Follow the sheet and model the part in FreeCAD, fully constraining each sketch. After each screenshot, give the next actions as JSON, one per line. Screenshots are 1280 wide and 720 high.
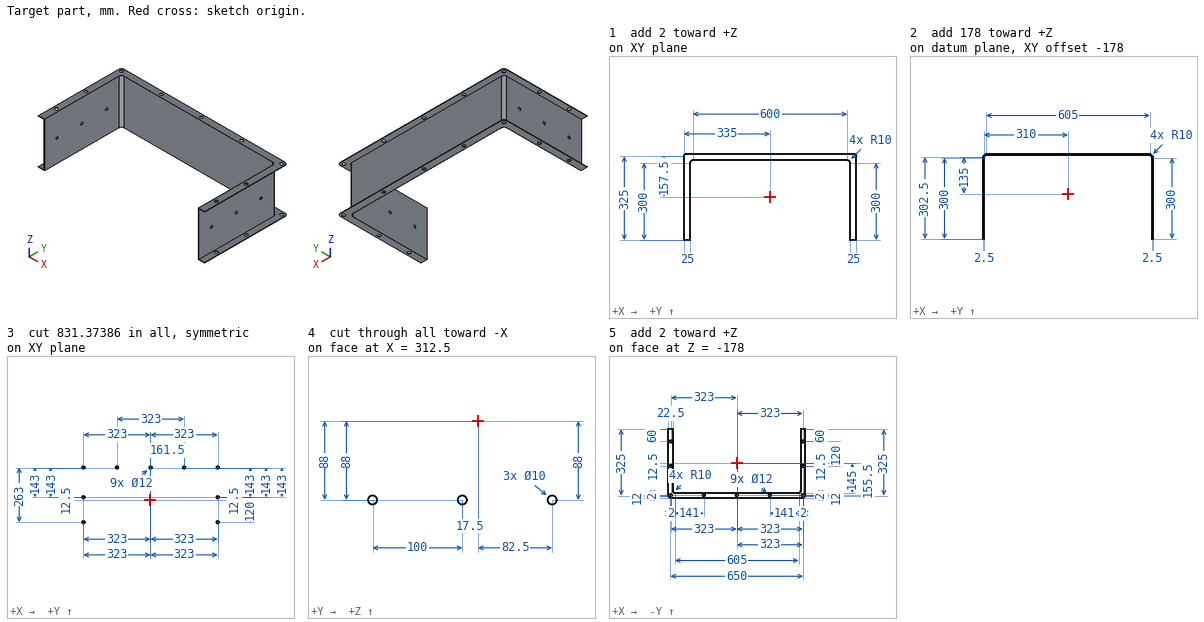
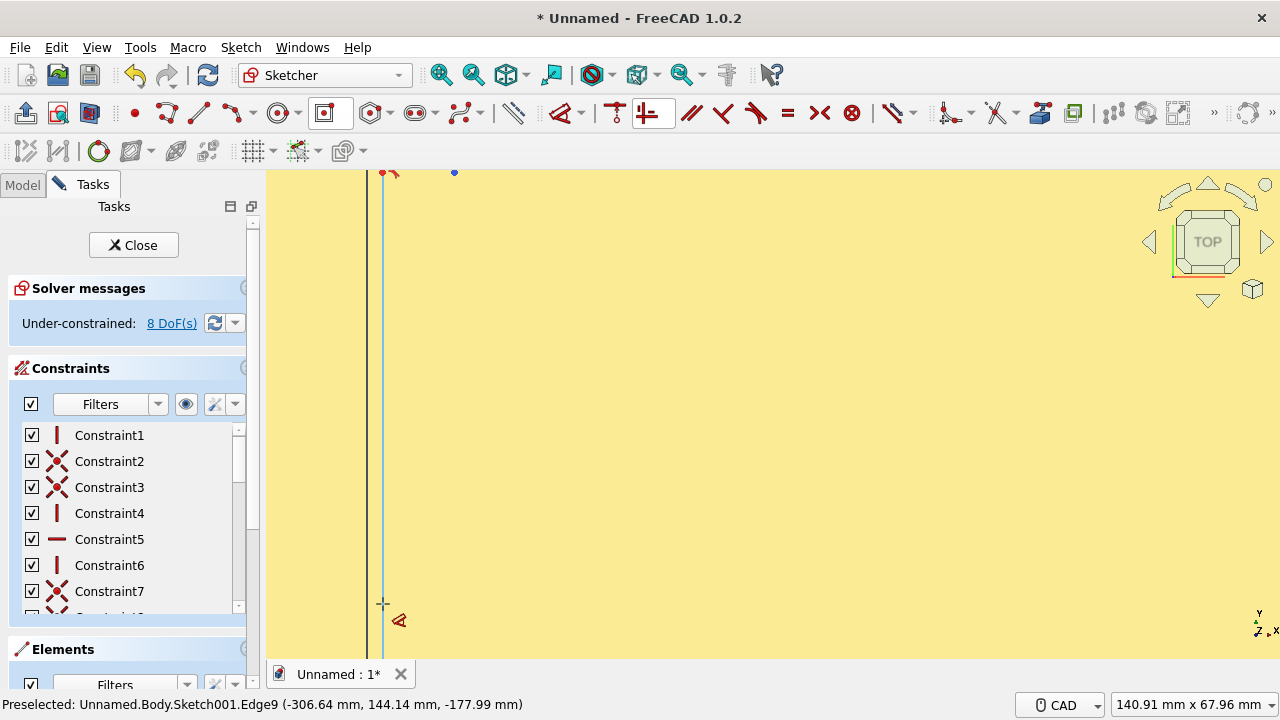
{"action": "left_click", "coordinate": [383, 603]}
{"action": "left_click", "coordinate": [349, 414]}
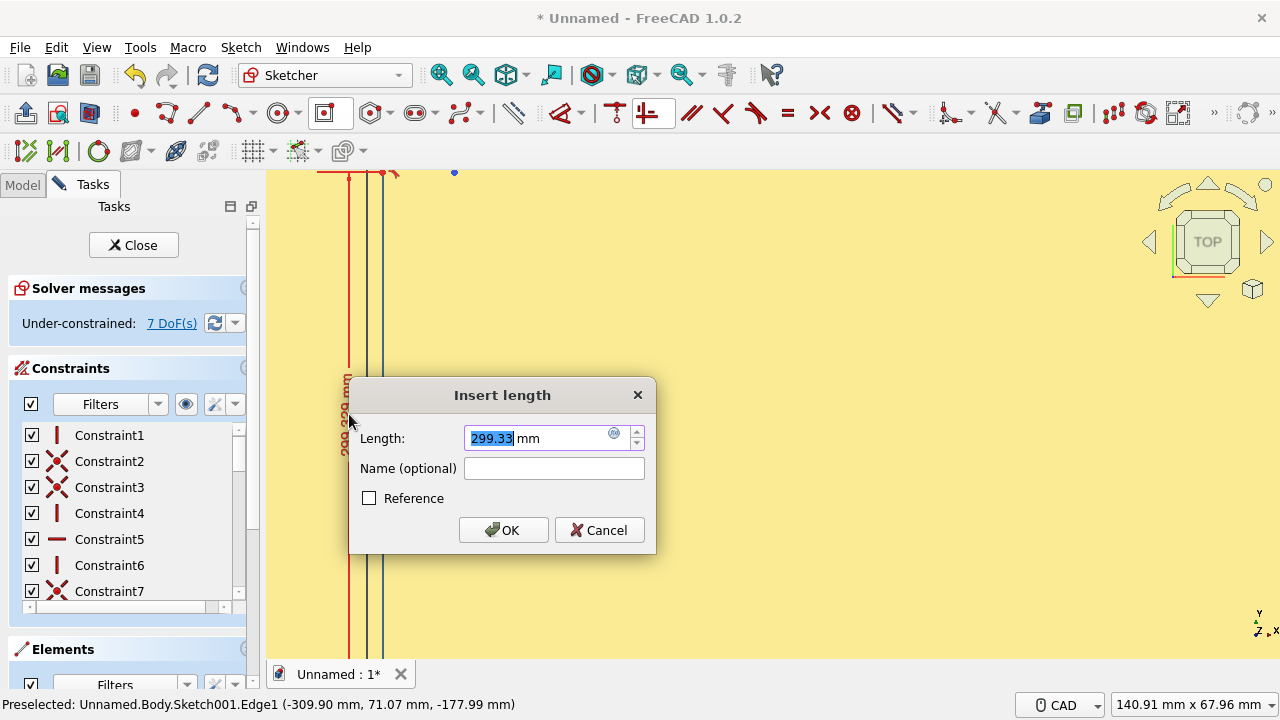
{"action": "type", "text": "300"}
{"action": "key", "text": "Return"}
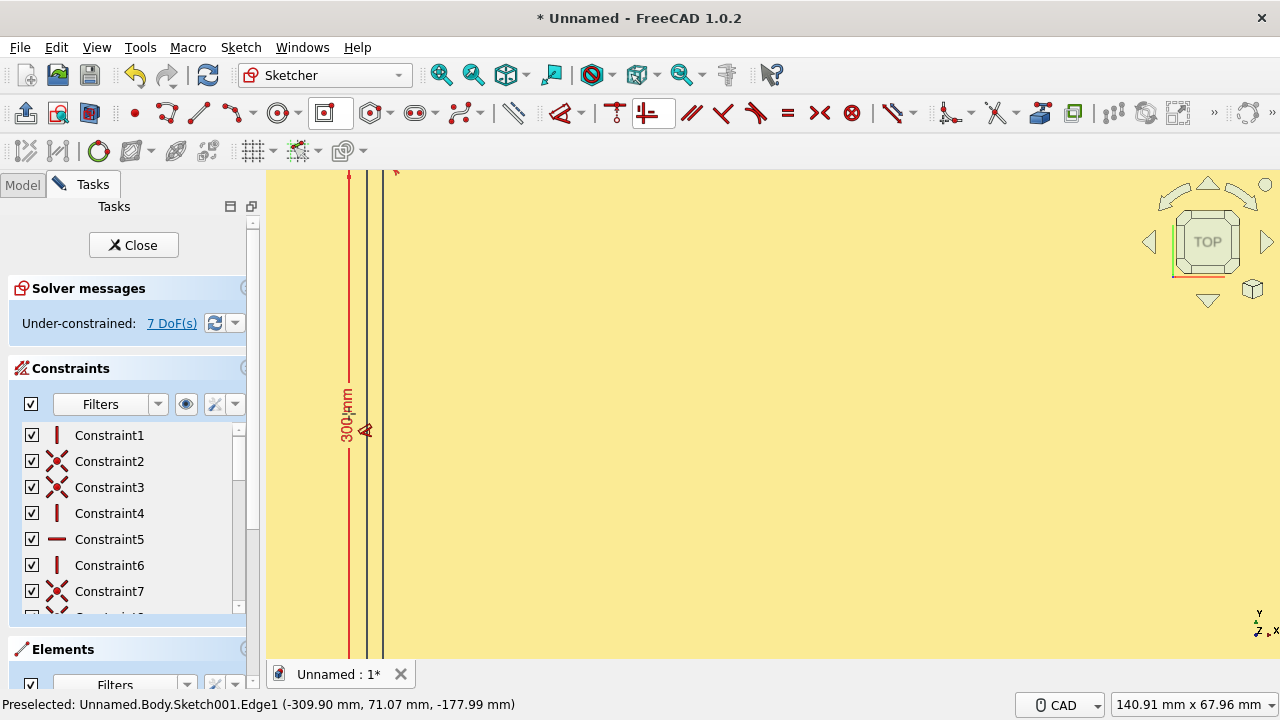
{"action": "scroll", "coordinate": [406, 292], "scroll_direction": "down", "scroll_amount": 10}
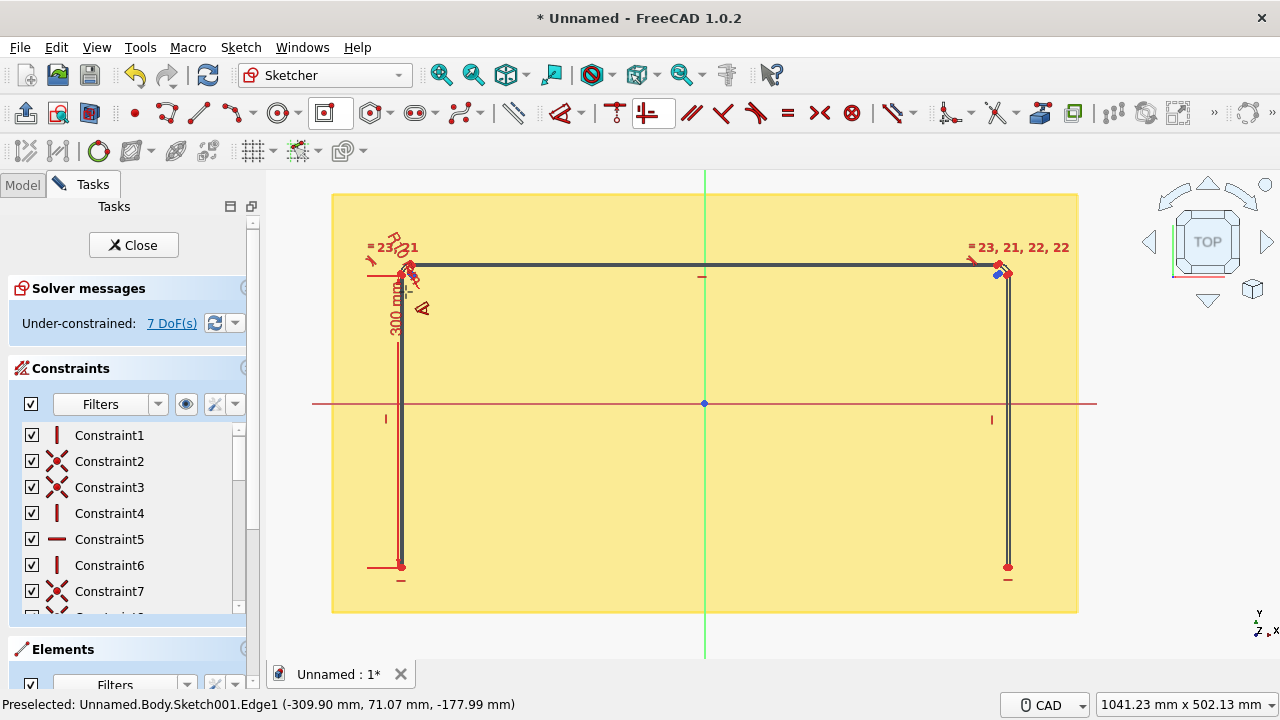
{"action": "scroll", "coordinate": [402, 568], "scroll_direction": "up", "scroll_amount": 14}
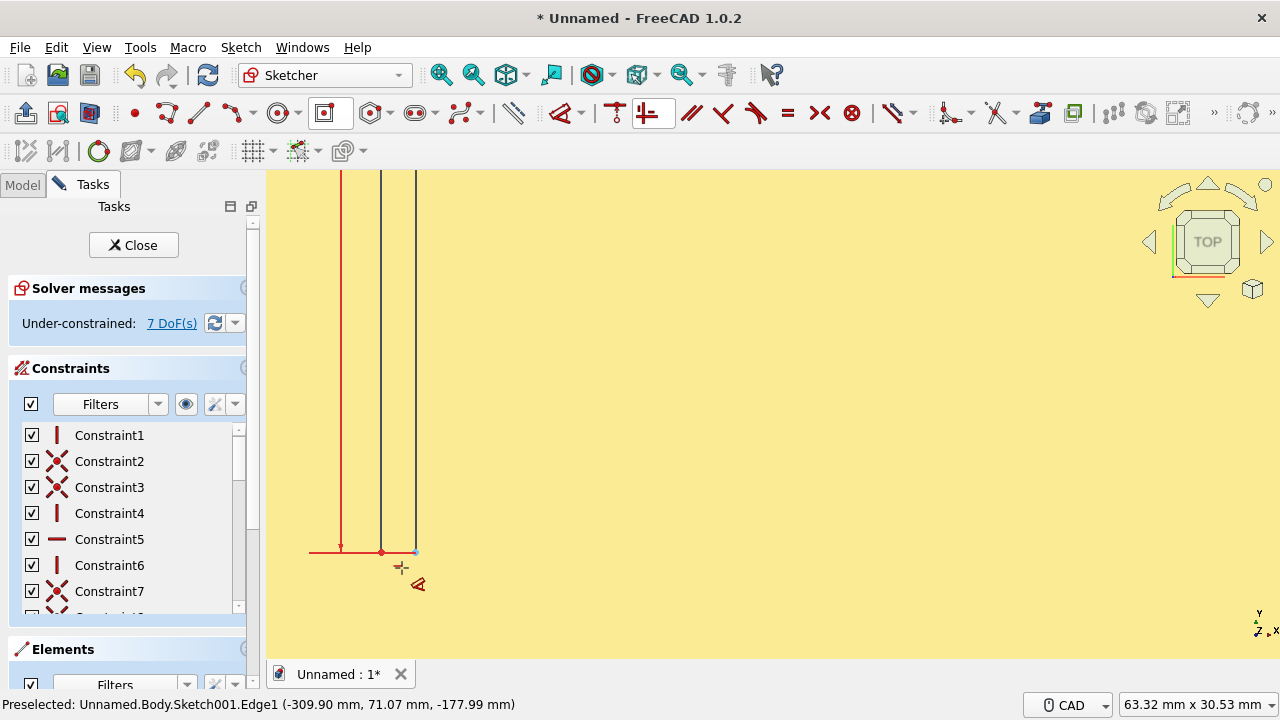
{"action": "left_click", "coordinate": [399, 553]}
{"action": "left_click", "coordinate": [399, 587]}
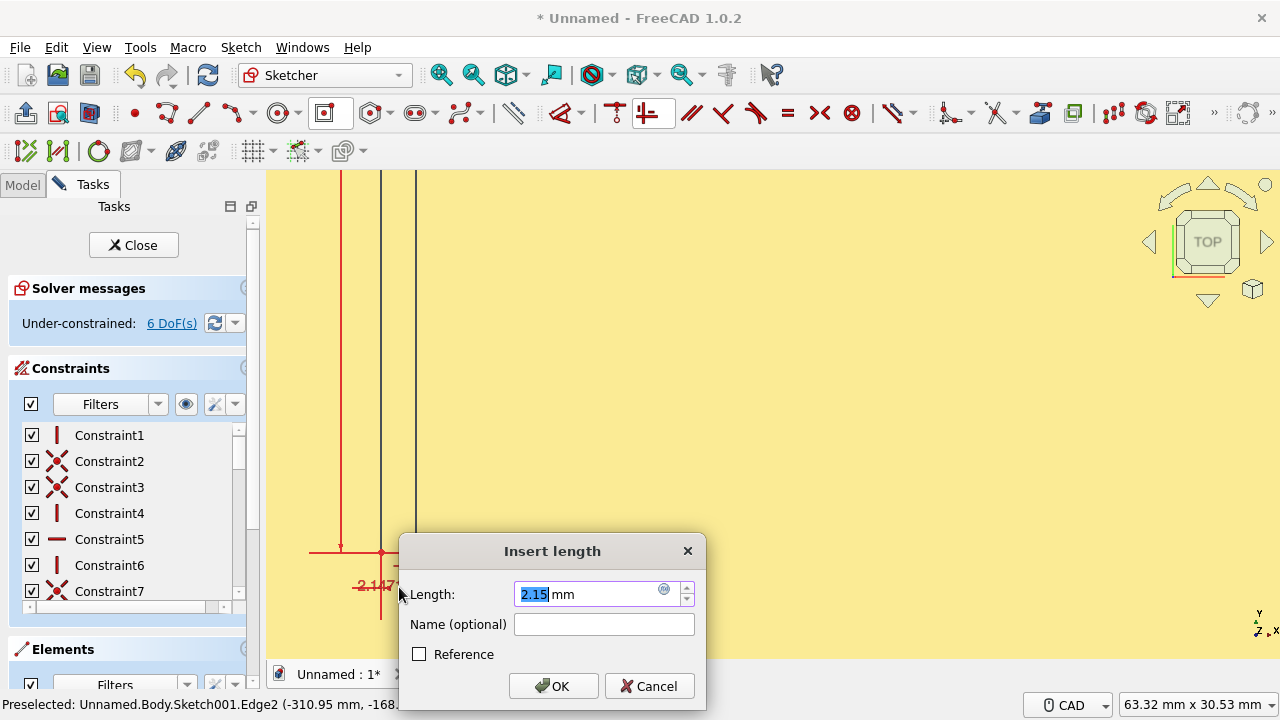
{"action": "type", "text": "2.5"}
{"action": "key", "text": "Return"}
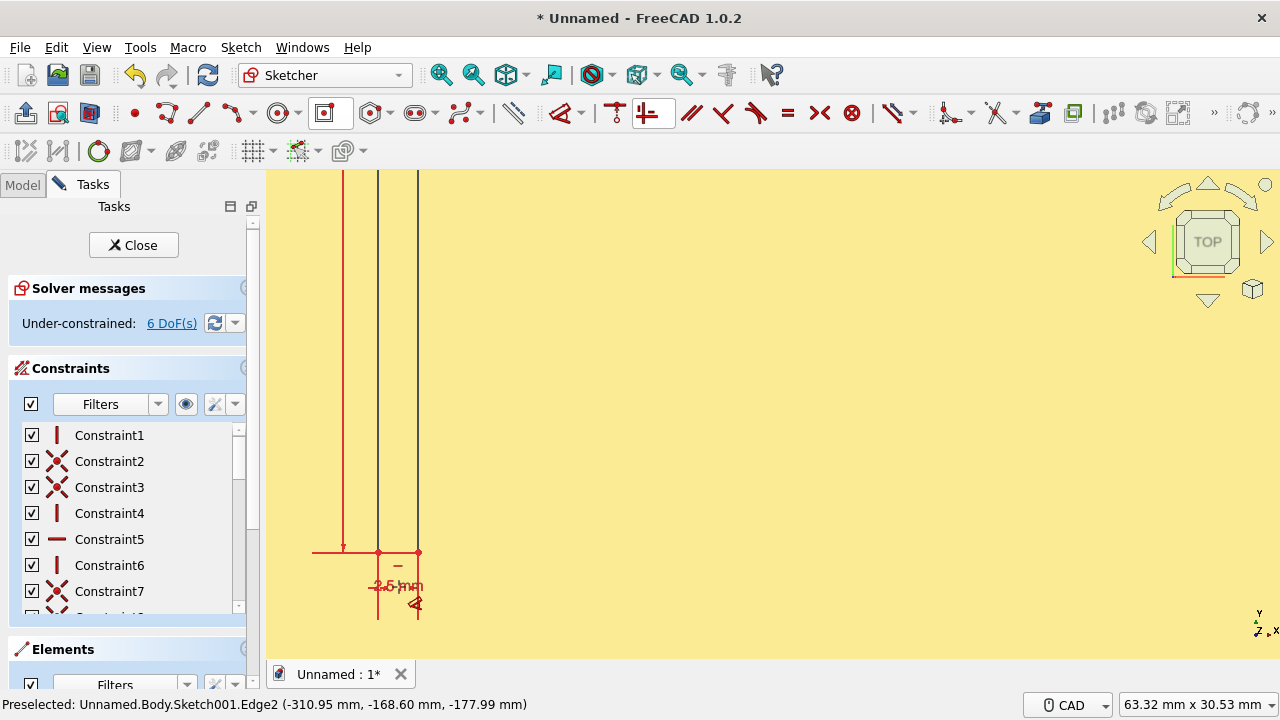
{"action": "scroll", "coordinate": [402, 569], "scroll_direction": "down", "scroll_amount": 14}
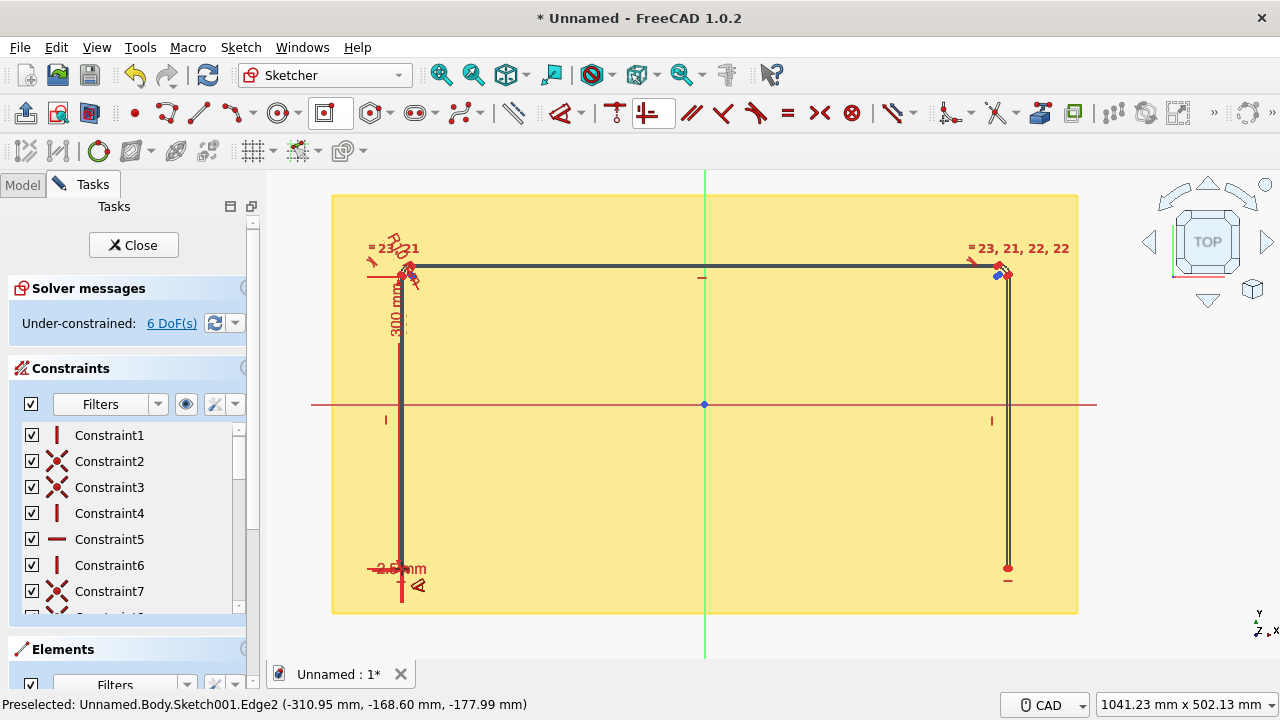
{"action": "scroll", "coordinate": [587, 265], "scroll_direction": "up", "scroll_amount": 10}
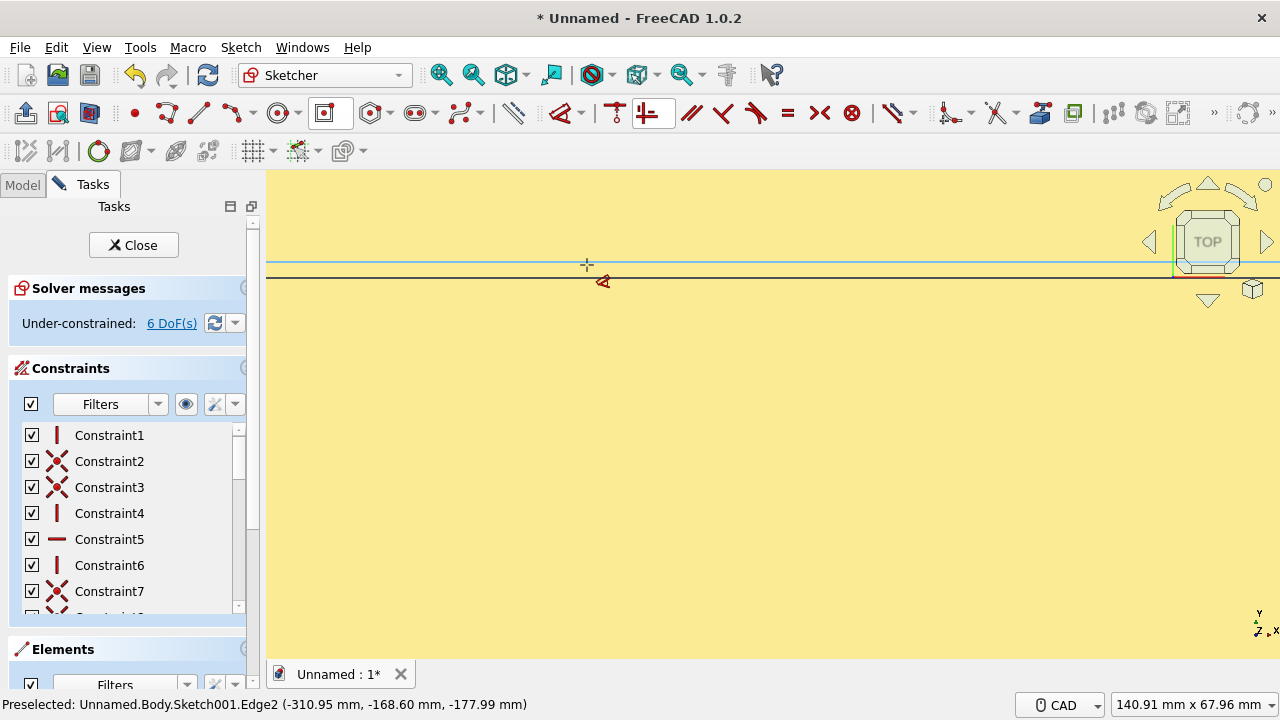
{"action": "left_click", "coordinate": [587, 262]}
{"action": "left_click", "coordinate": [704, 228]}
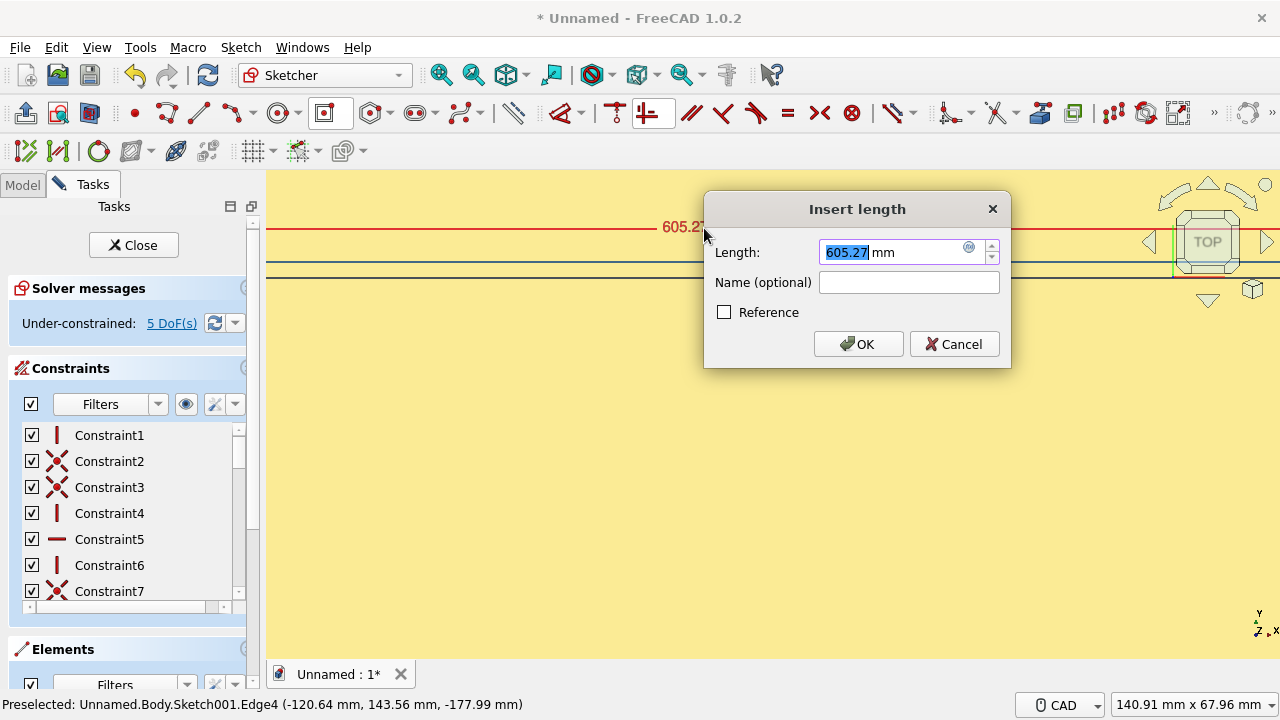
{"action": "type", "text": "605"}
{"action": "key", "text": "Return"}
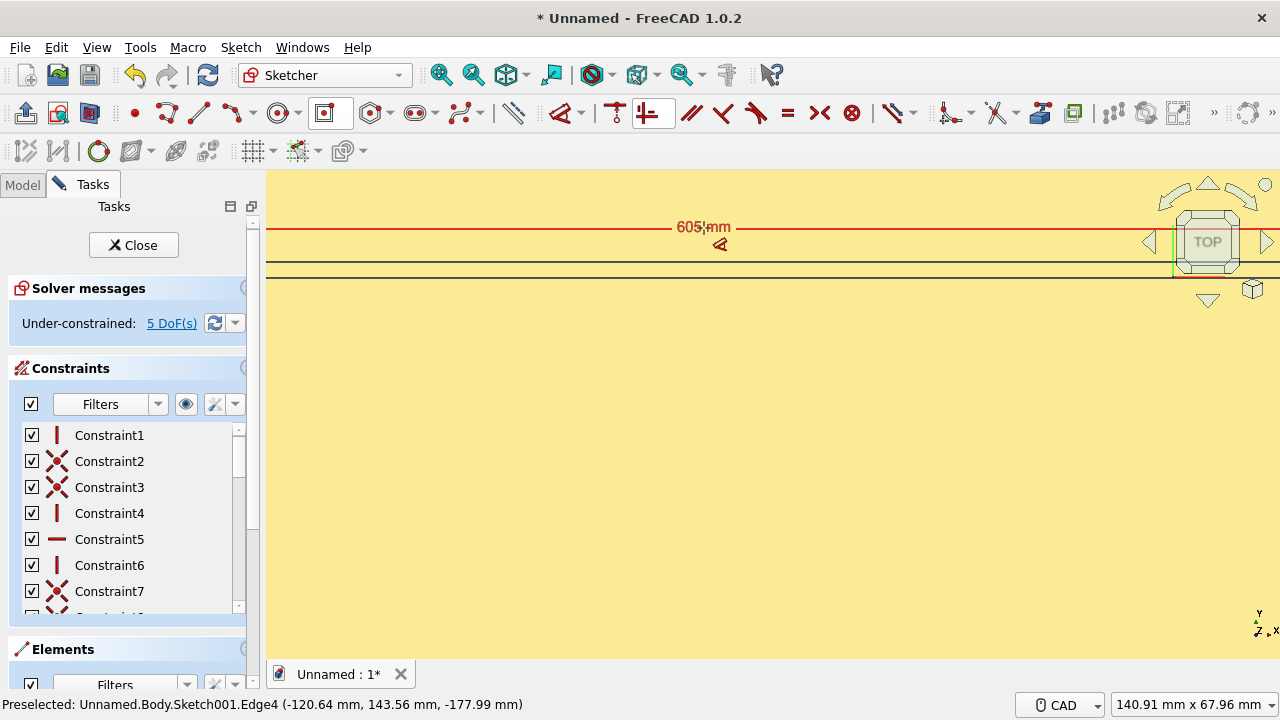
{"action": "scroll", "coordinate": [587, 264], "scroll_direction": "down", "scroll_amount": 10}